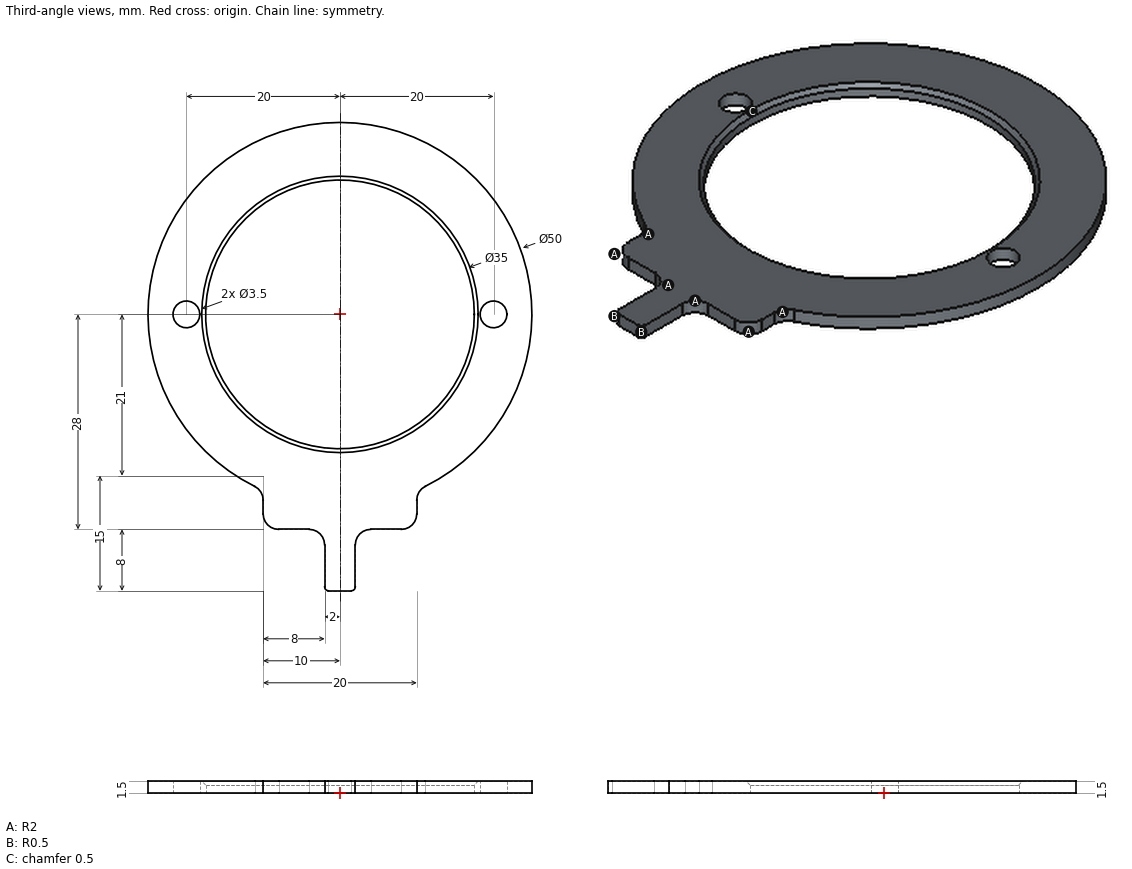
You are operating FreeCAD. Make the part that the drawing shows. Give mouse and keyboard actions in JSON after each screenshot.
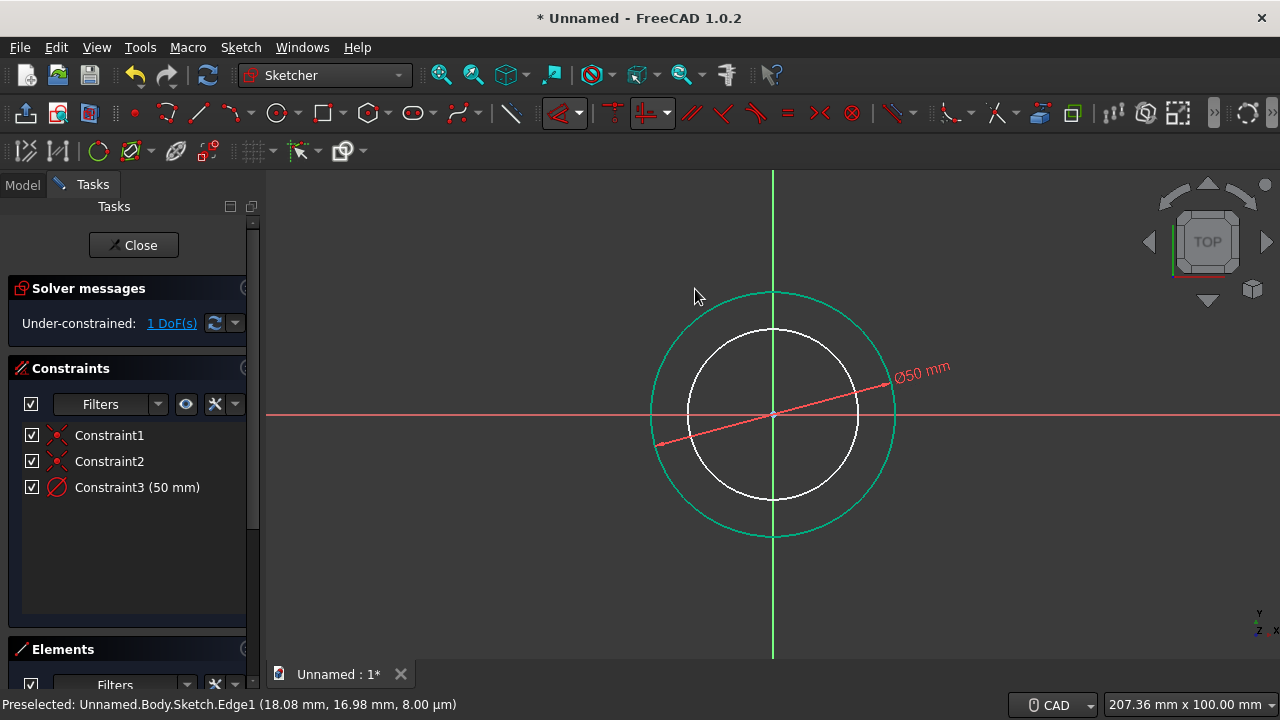
{"action": "left_click", "coordinate": [833, 354]}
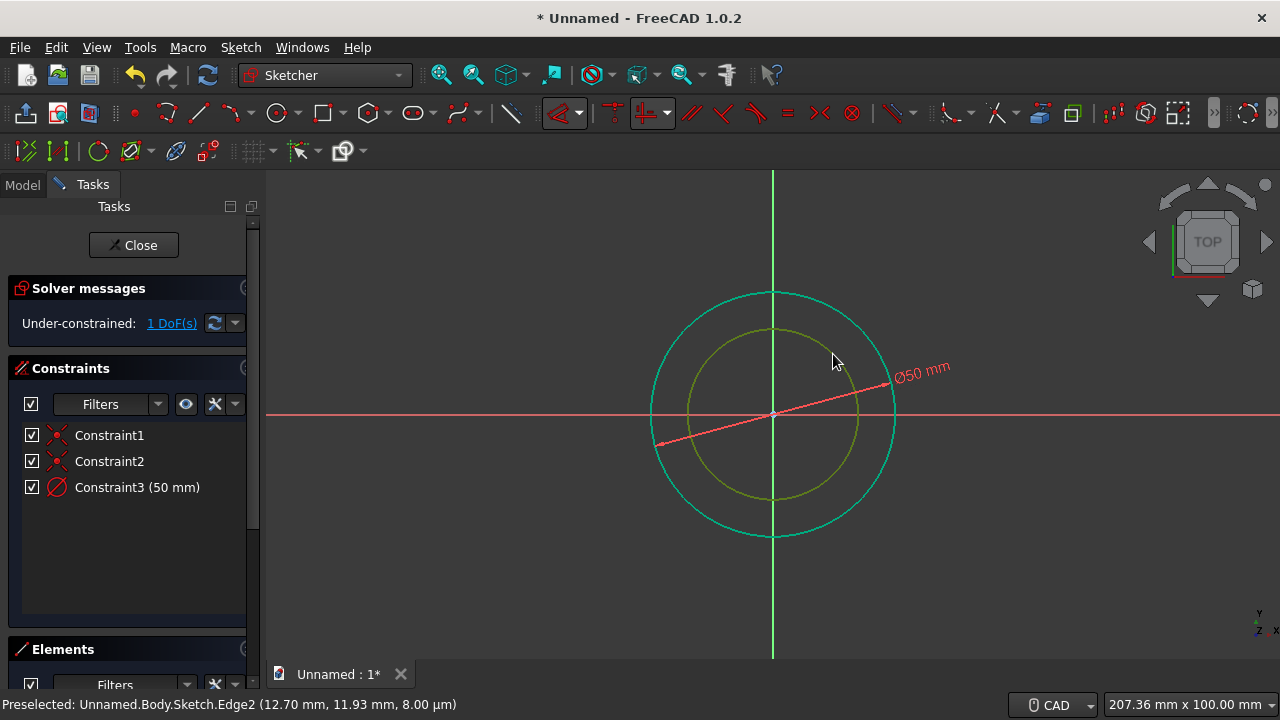
{"action": "left_click", "coordinate": [582, 114]}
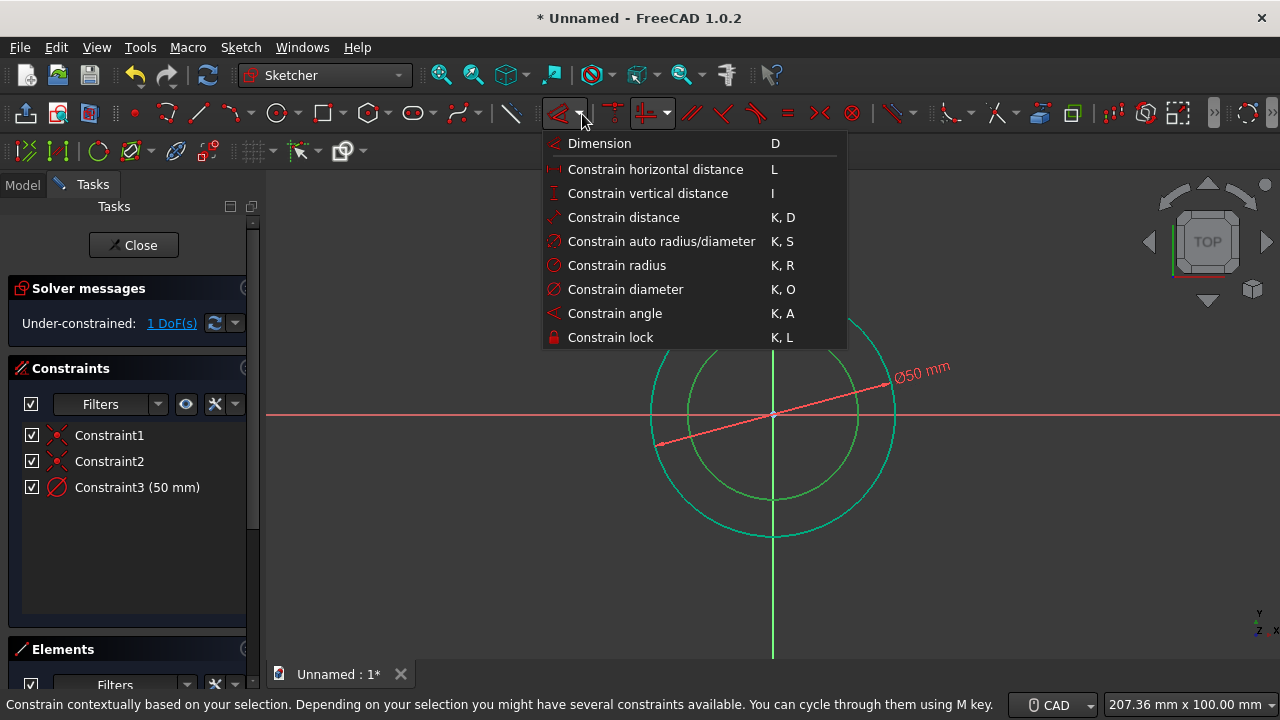
{"action": "left_click", "coordinate": [695, 289]}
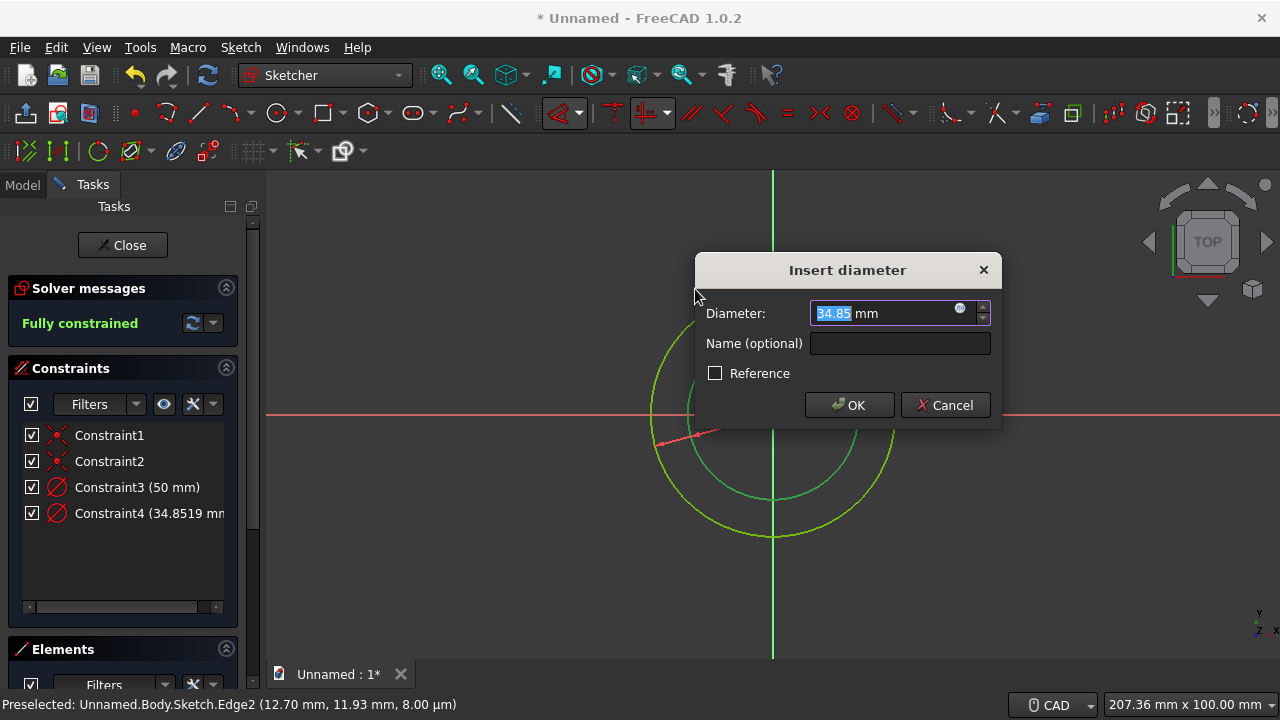
{"action": "type", "text": "35"}
{"action": "key", "text": "Return"}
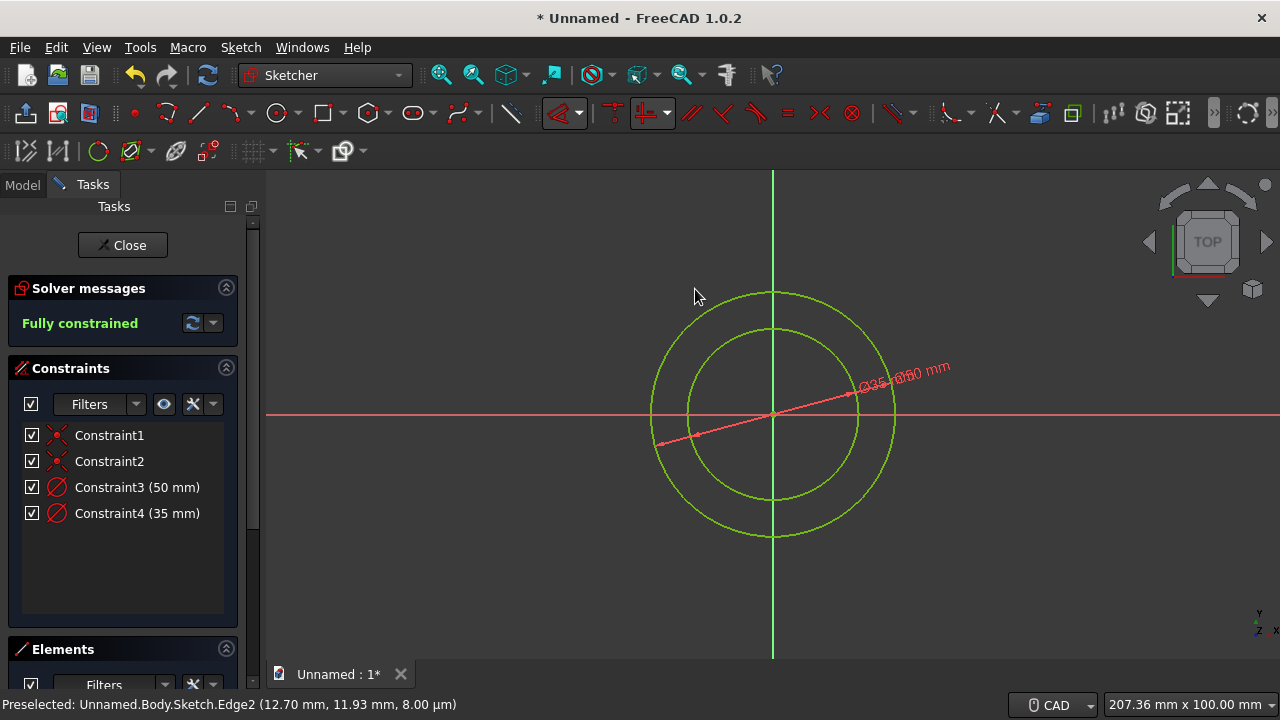
{"action": "left_click", "coordinate": [123, 245]}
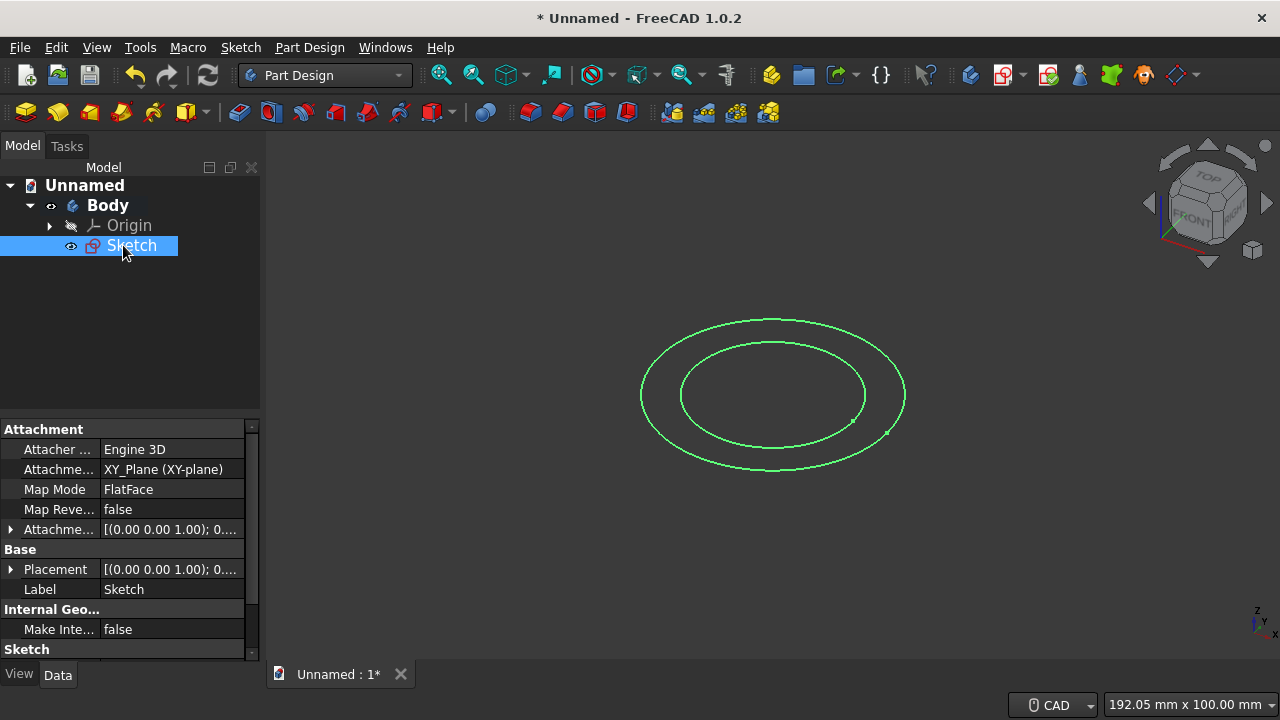
{"action": "left_click", "coordinate": [26, 112]}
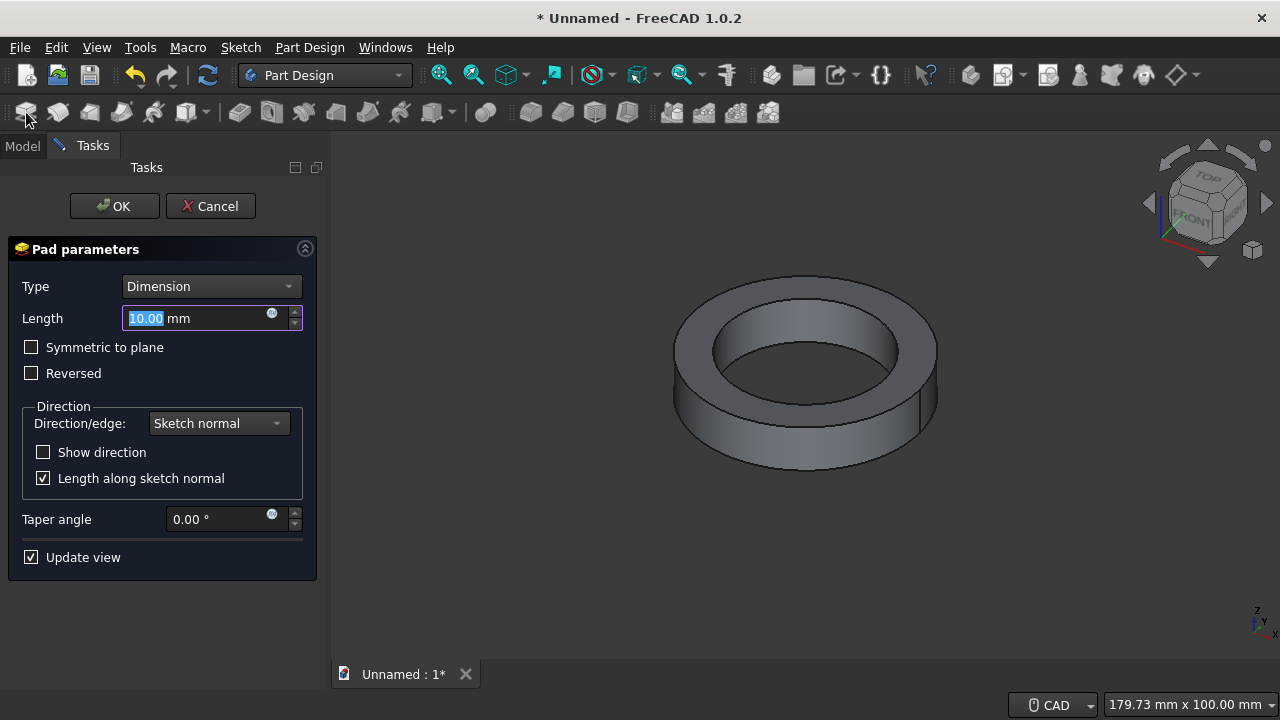
{"action": "type", "text": "1.5"}
{"action": "key", "text": "Tab"}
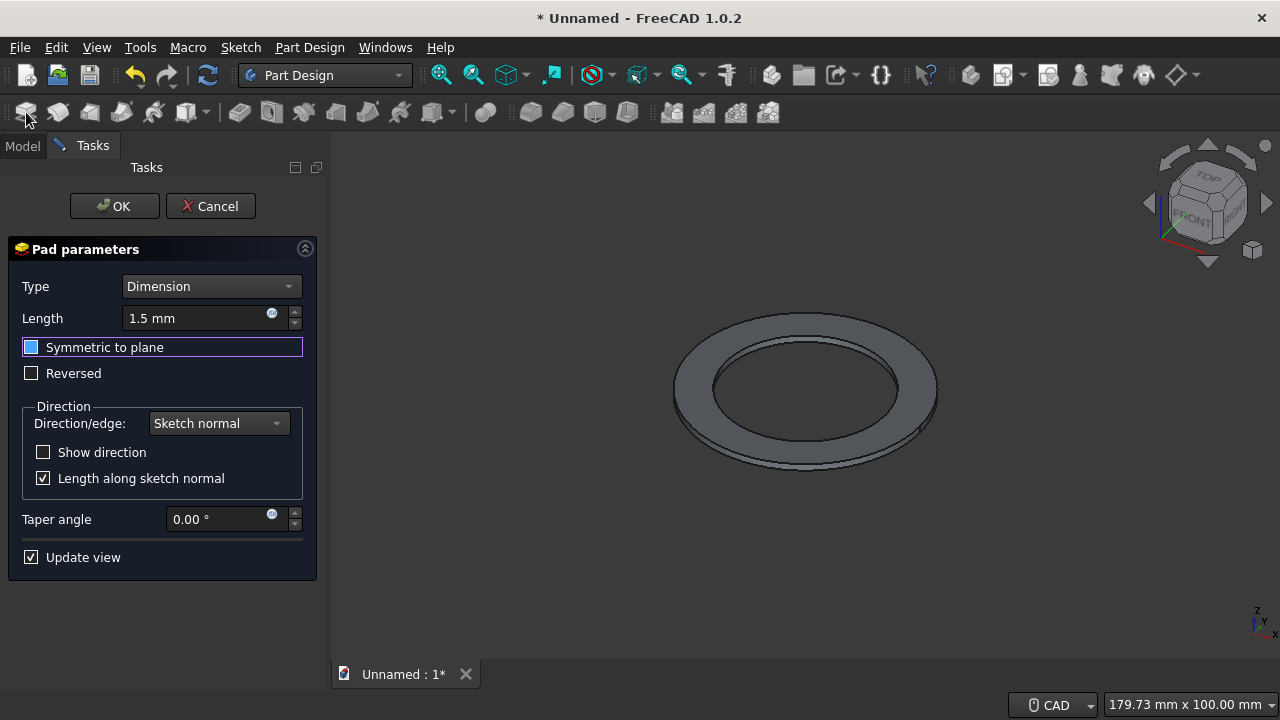
{"action": "left_click", "coordinate": [115, 206]}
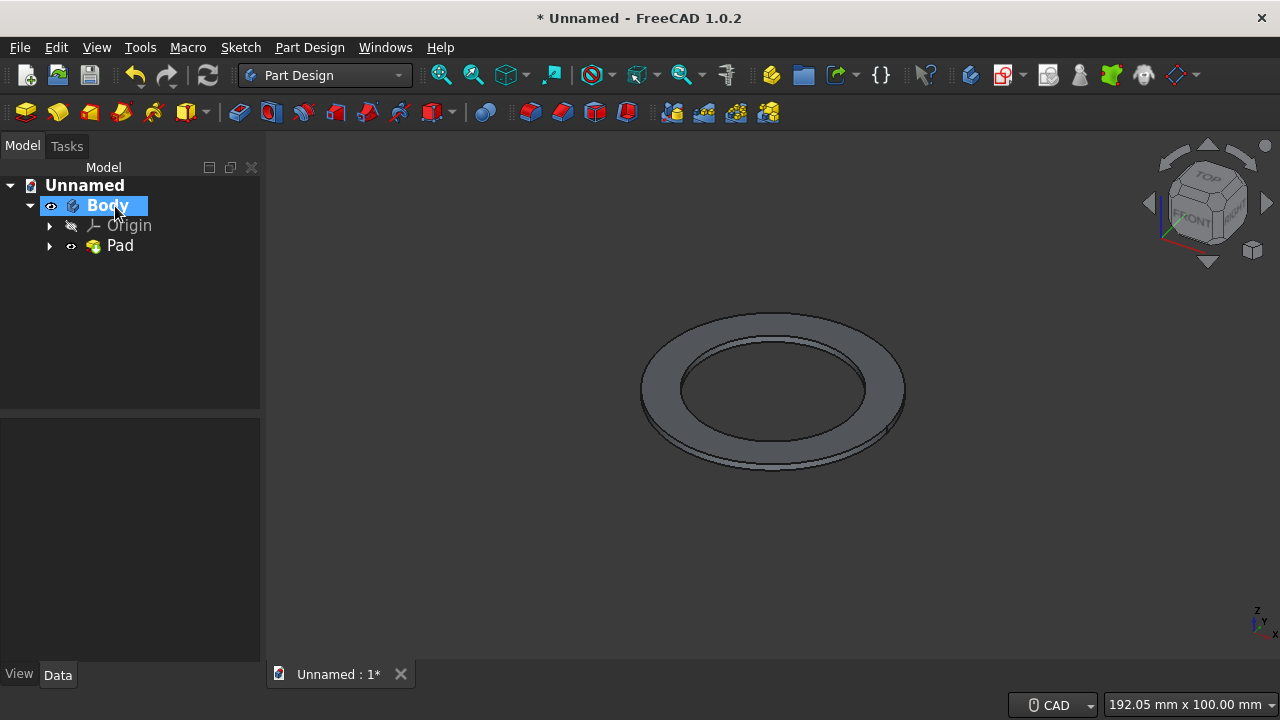
{"action": "left_click", "coordinate": [442, 76]}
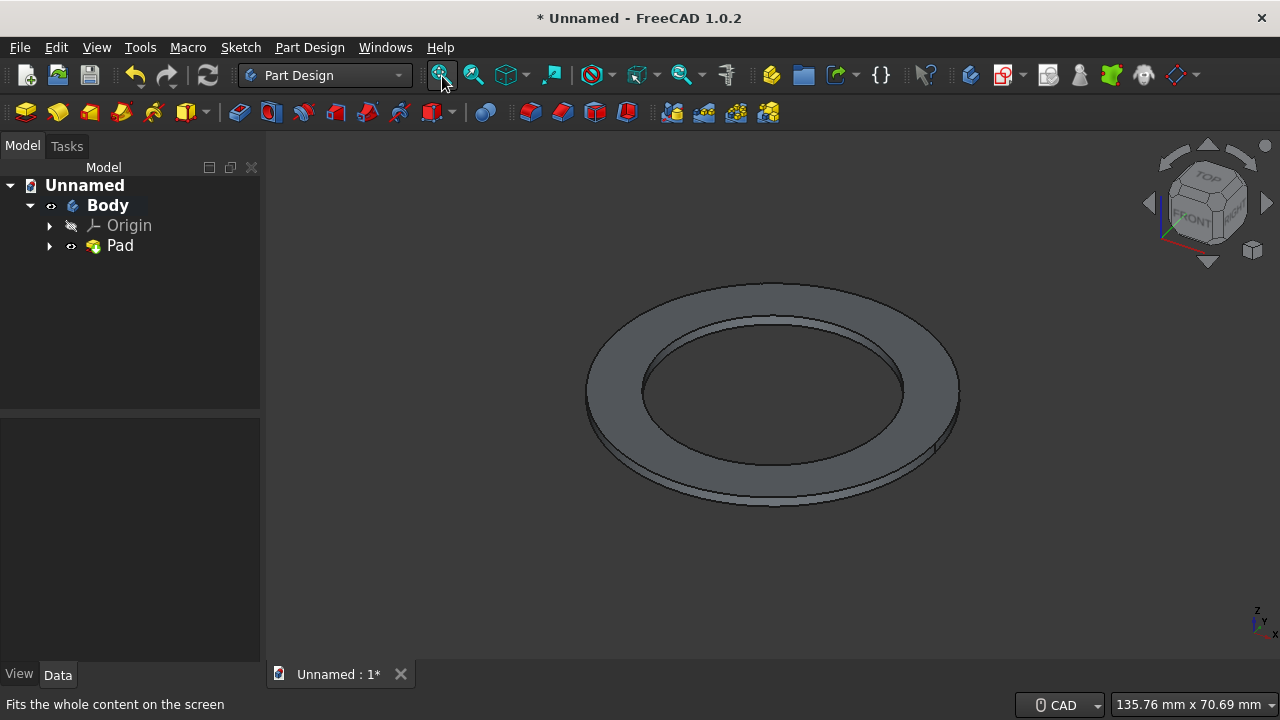
{"action": "left_click", "coordinate": [693, 469]}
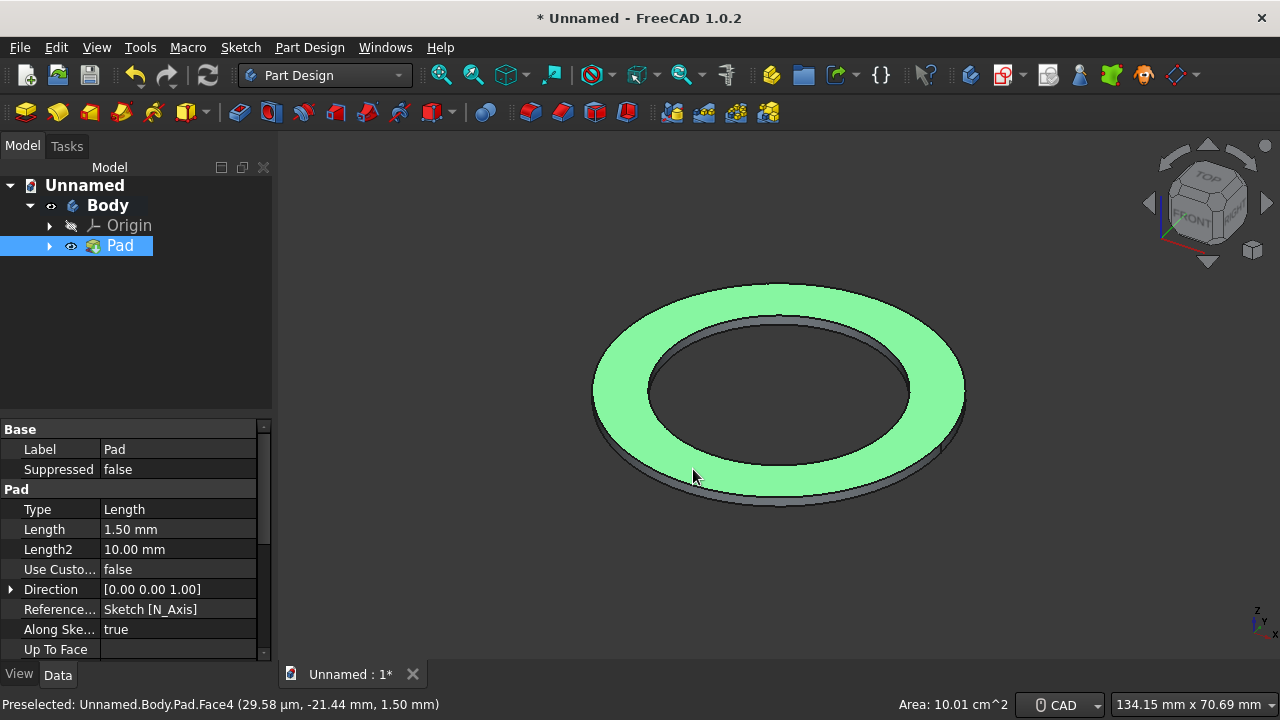
{"action": "left_click", "coordinate": [1004, 76]}